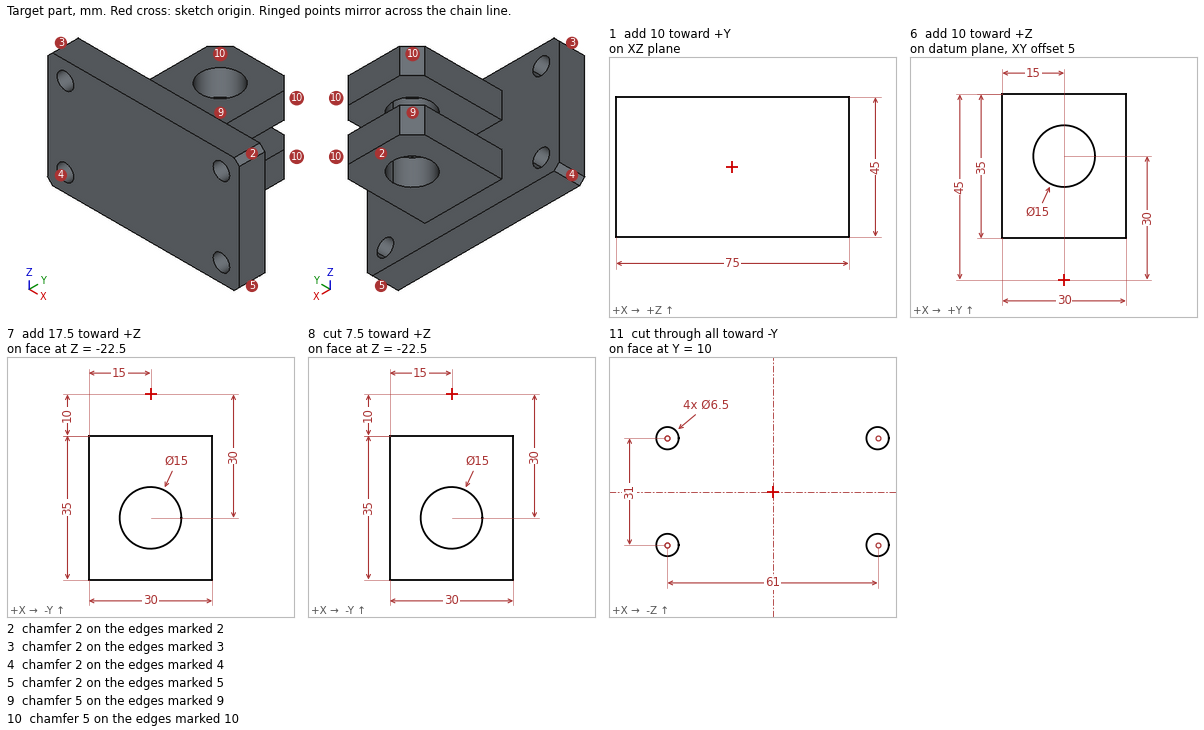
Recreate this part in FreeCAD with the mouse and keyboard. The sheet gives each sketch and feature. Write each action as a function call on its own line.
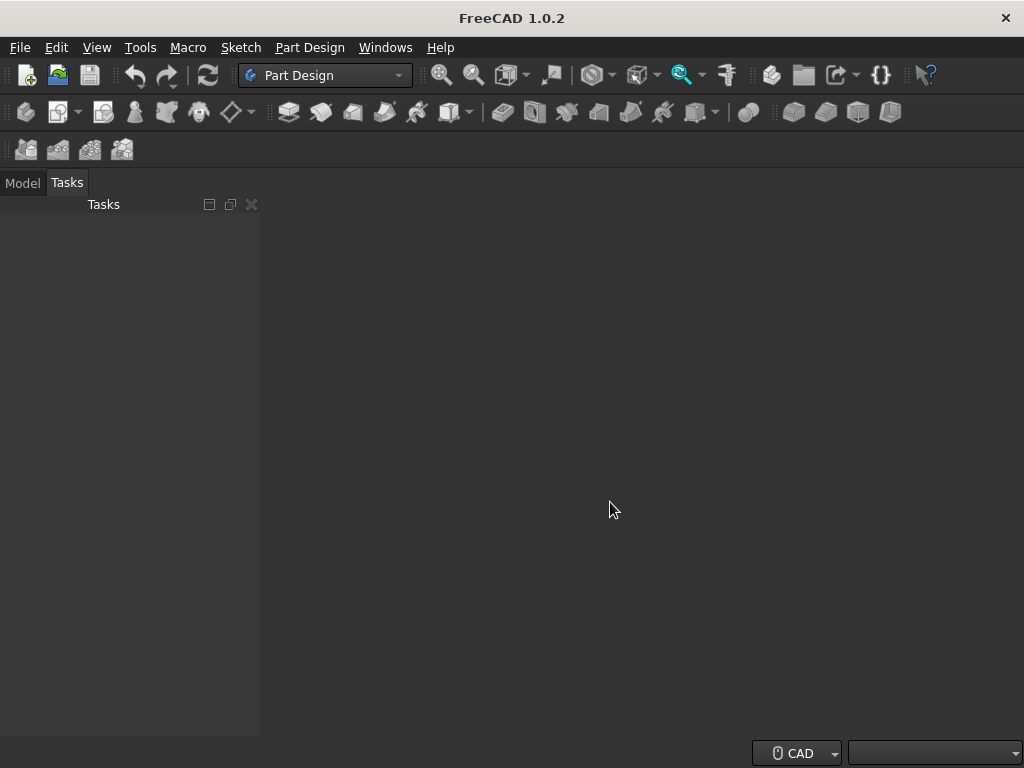
key(ctrl+n)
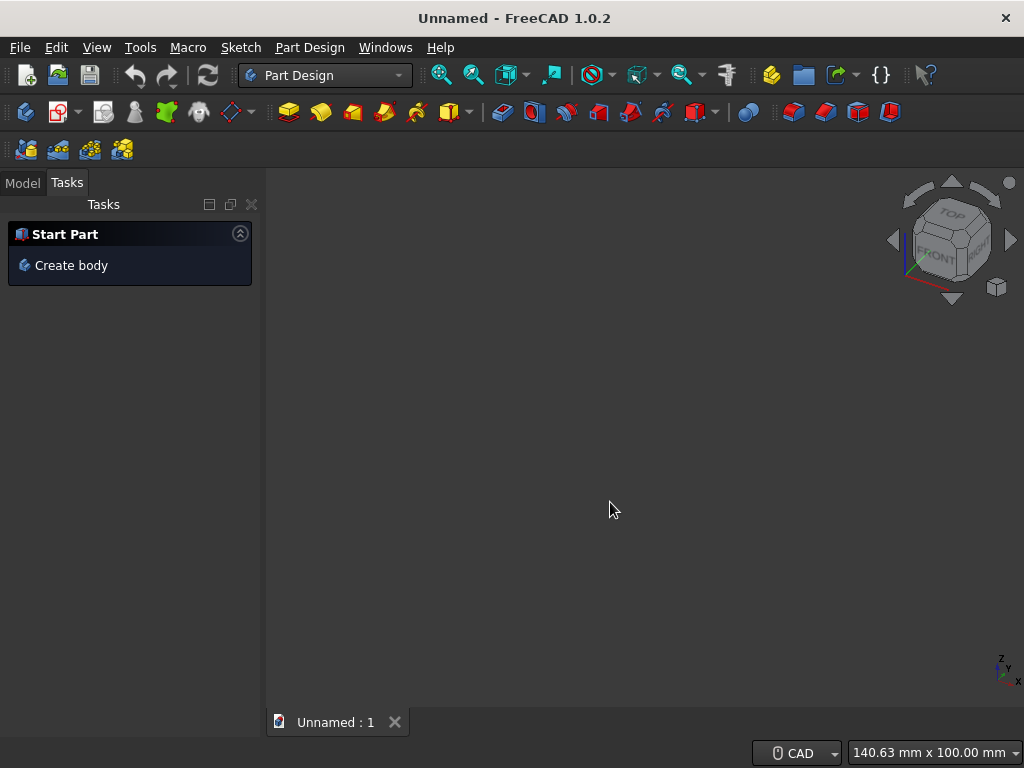
click(58, 112)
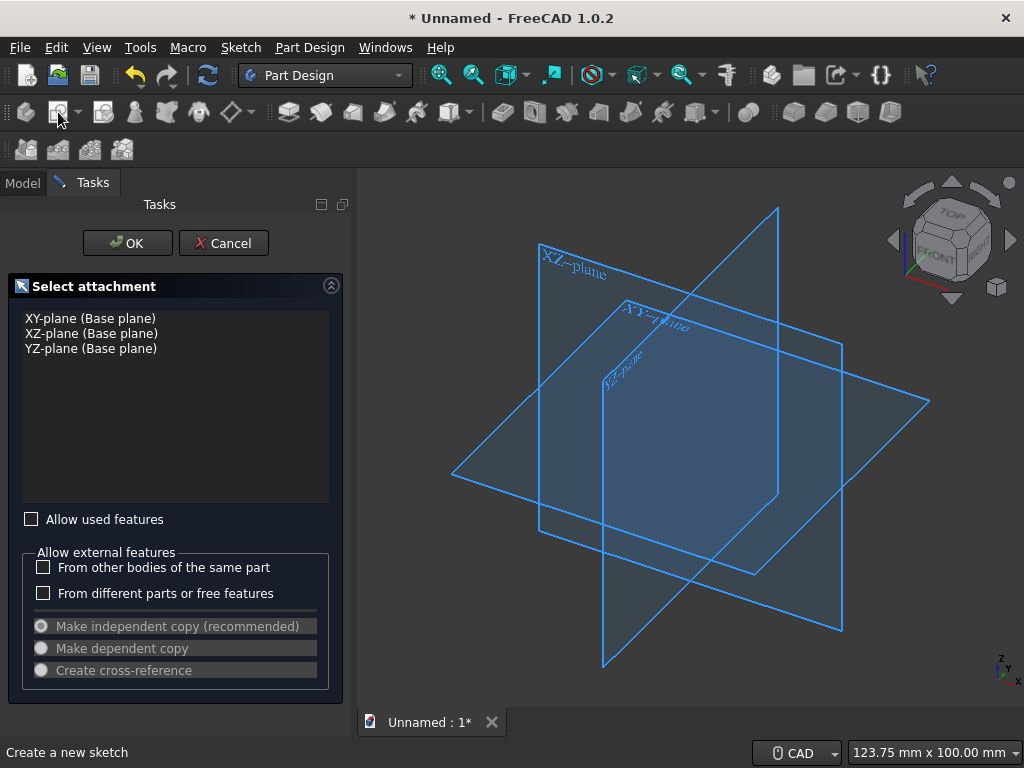
click(82, 334)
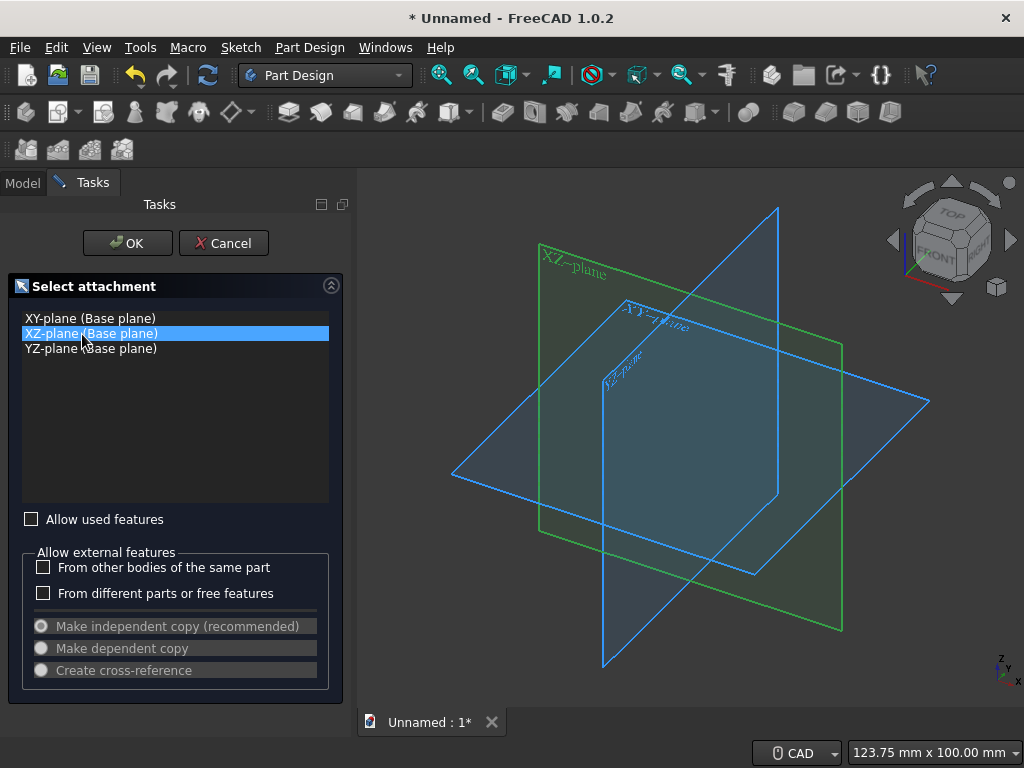
click(128, 243)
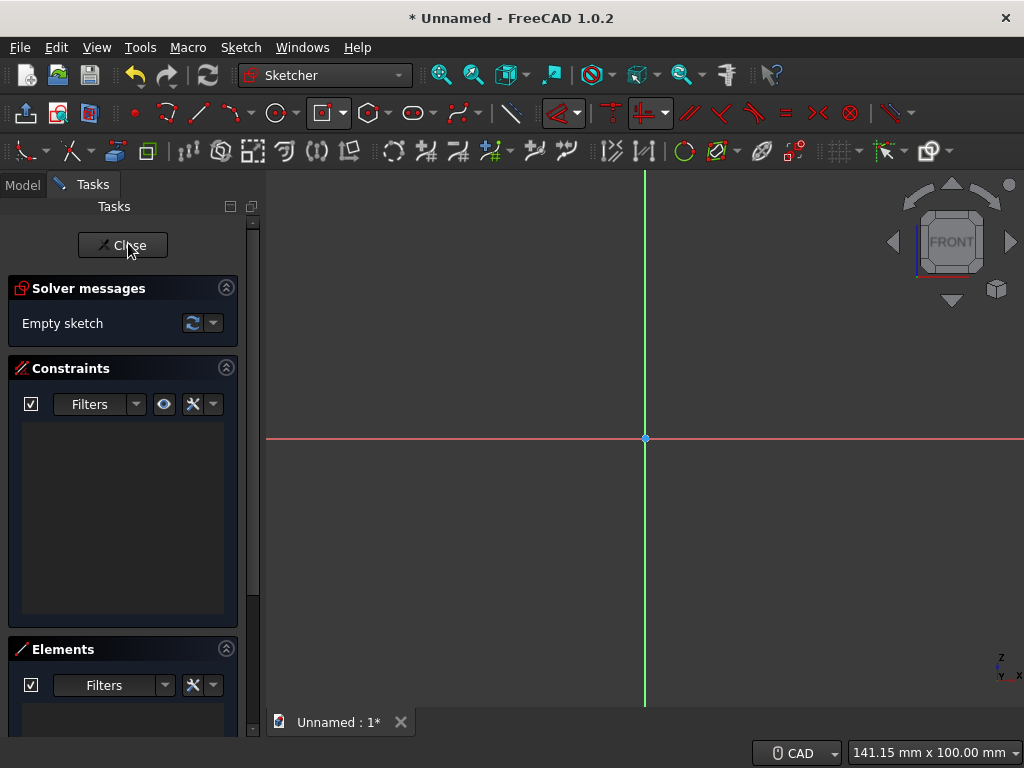
scroll(294, 439, down, 1)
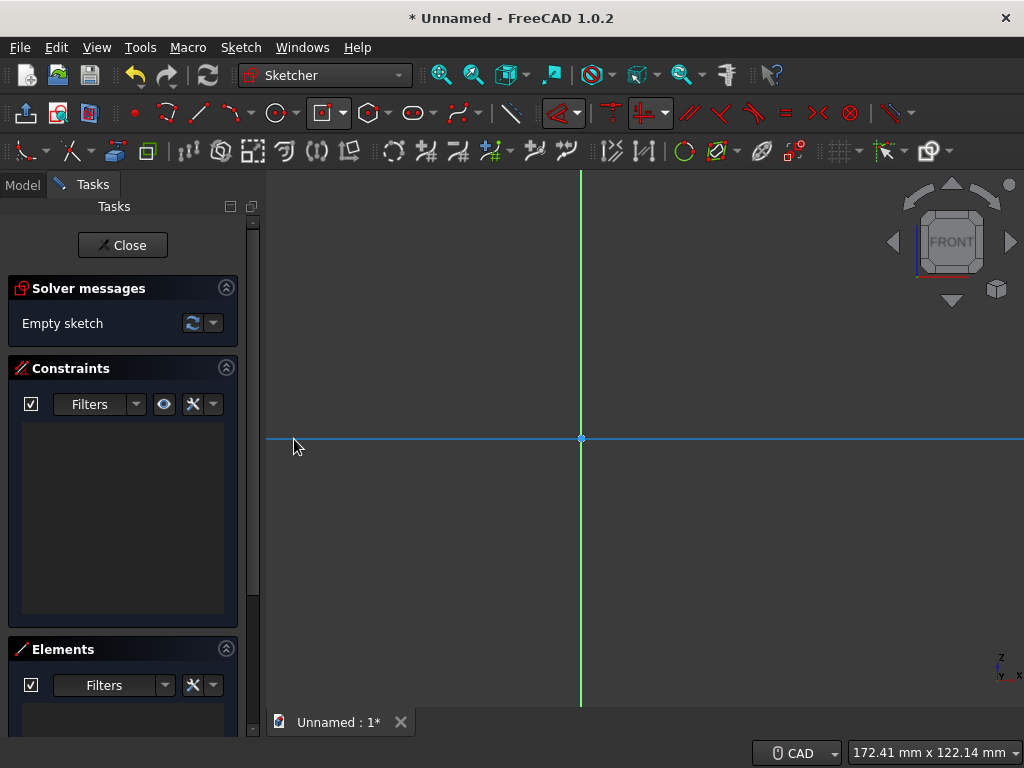
click(322, 114)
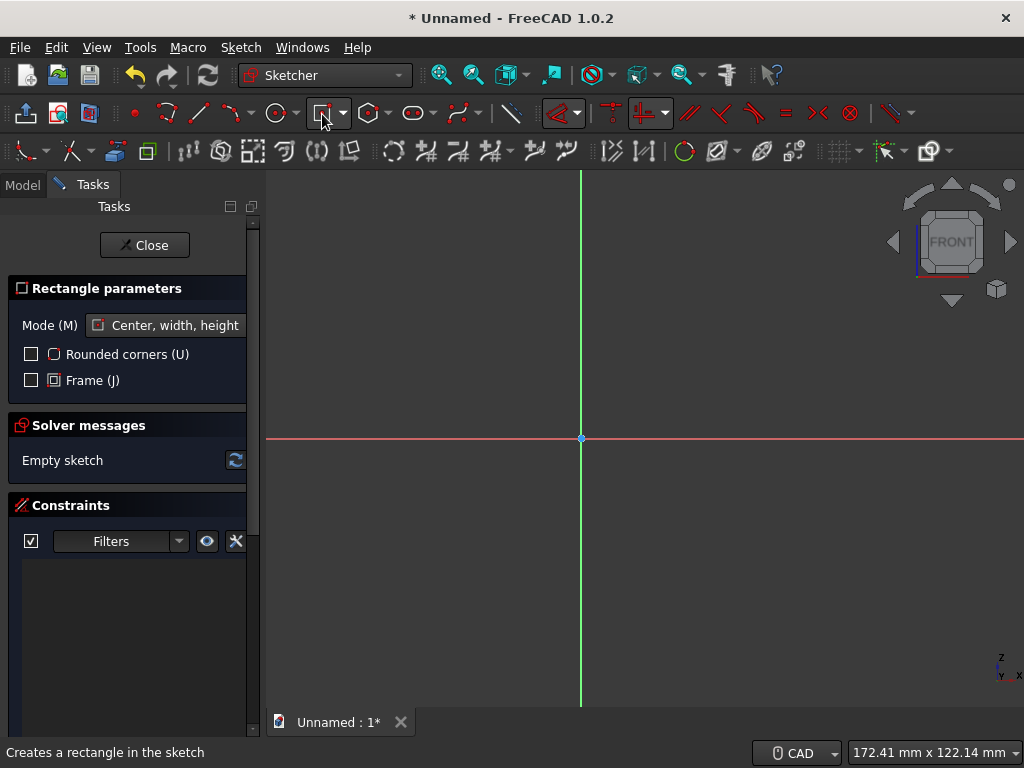
click(581, 439)
click(746, 340)
key(Escape)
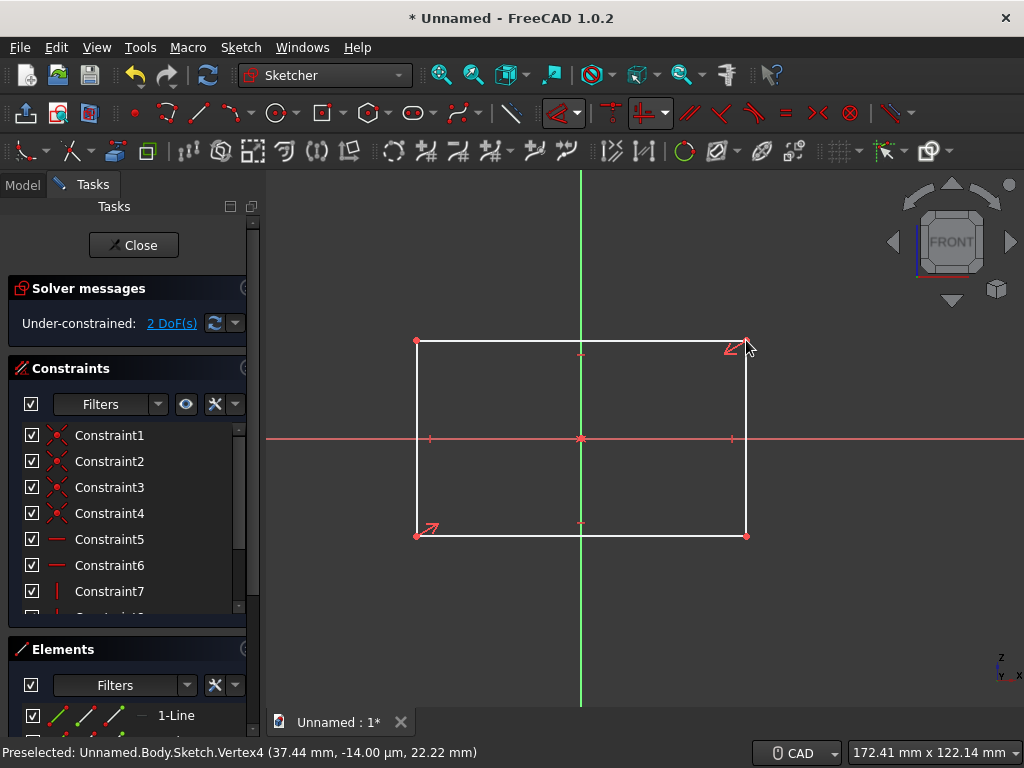
key(d)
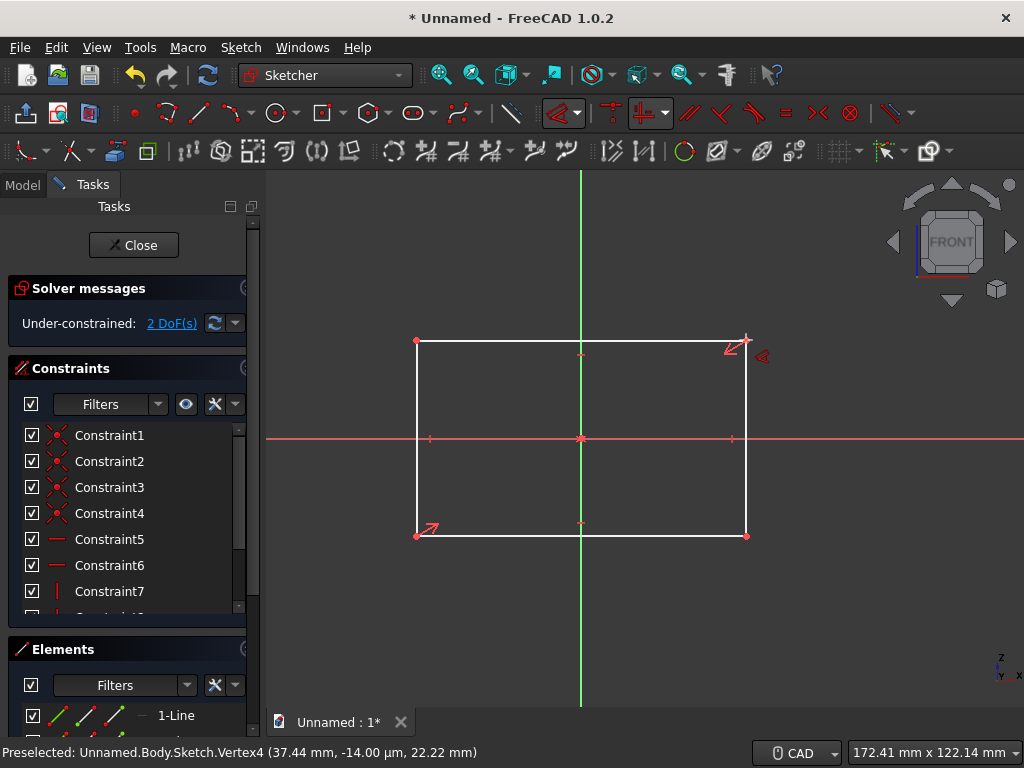
click(516, 536)
click(506, 570)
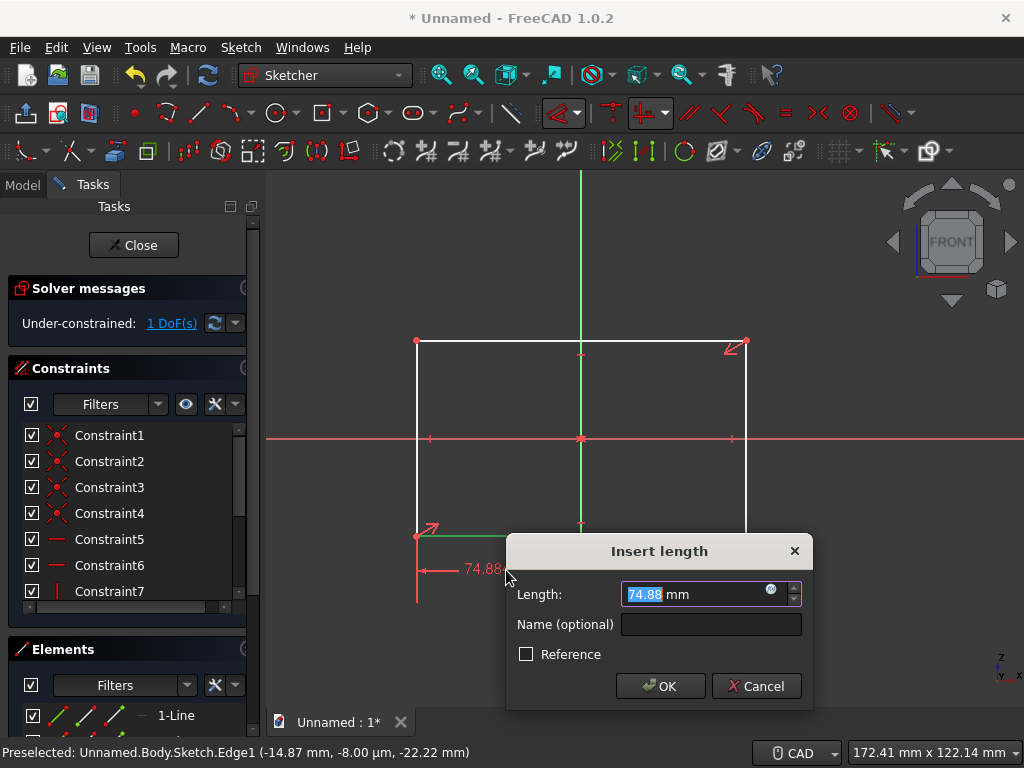
text(75)
key(Return)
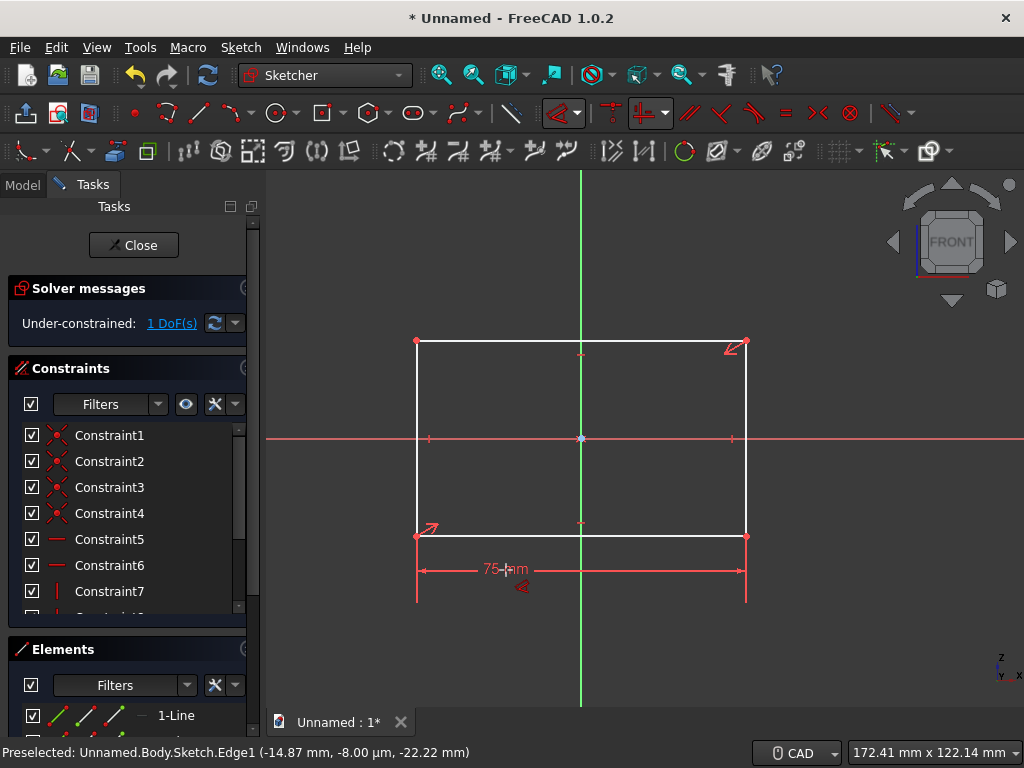
click(746, 478)
click(780, 394)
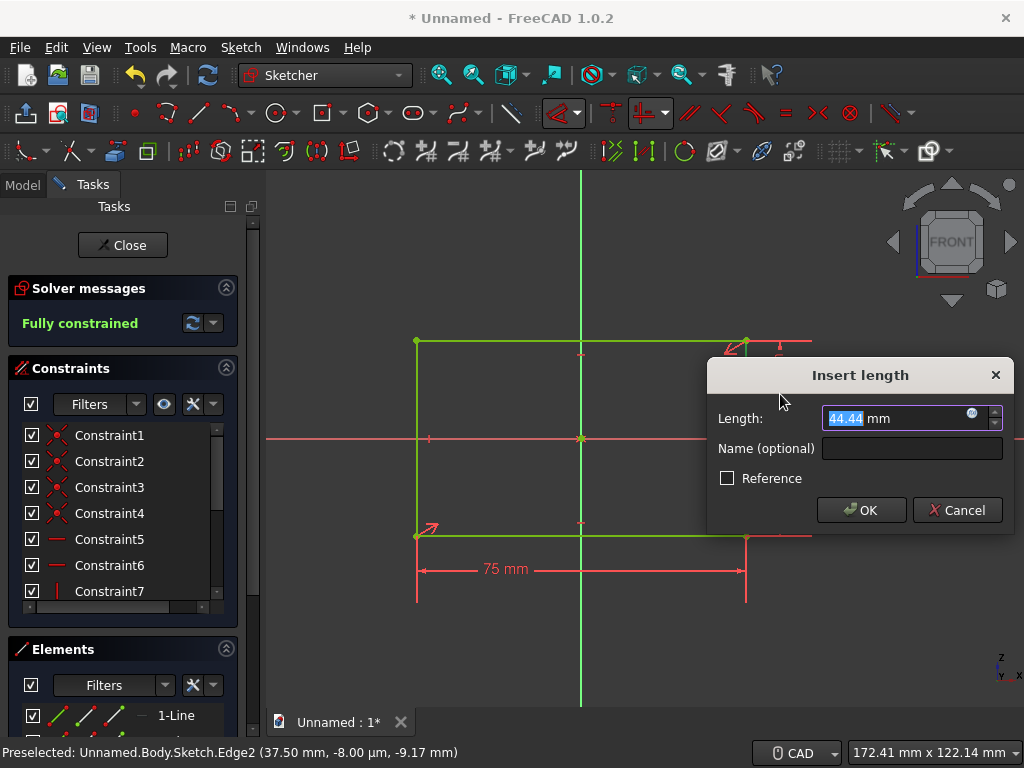
text(45)
key(Return)
key(Escape)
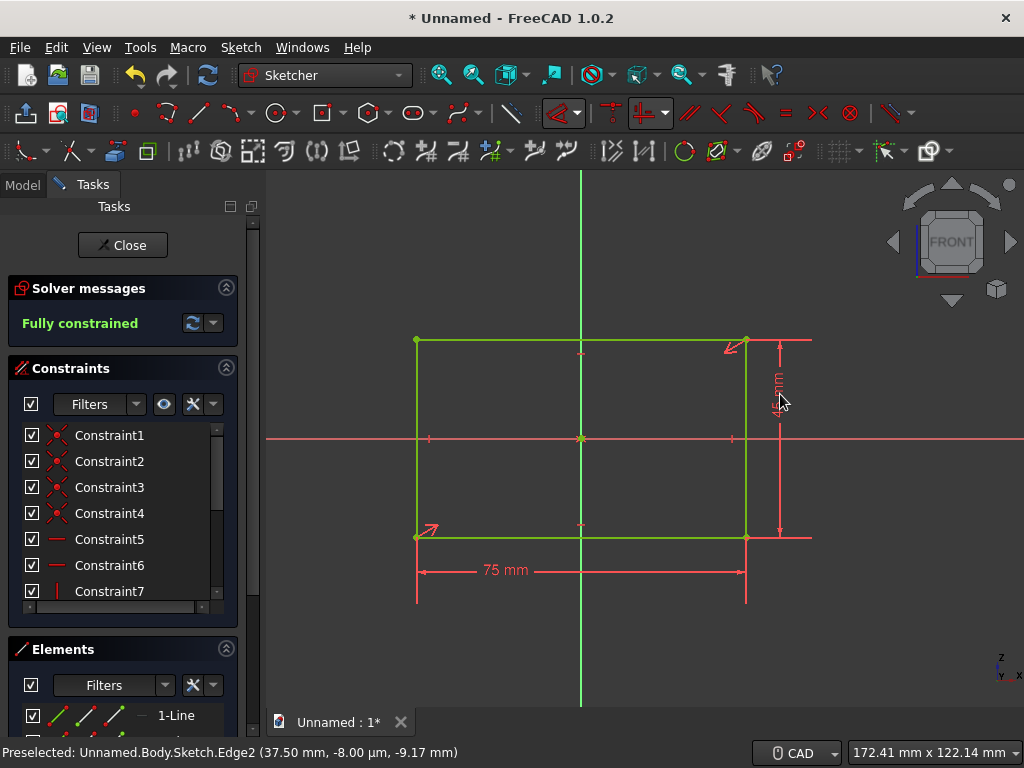
click(123, 245)